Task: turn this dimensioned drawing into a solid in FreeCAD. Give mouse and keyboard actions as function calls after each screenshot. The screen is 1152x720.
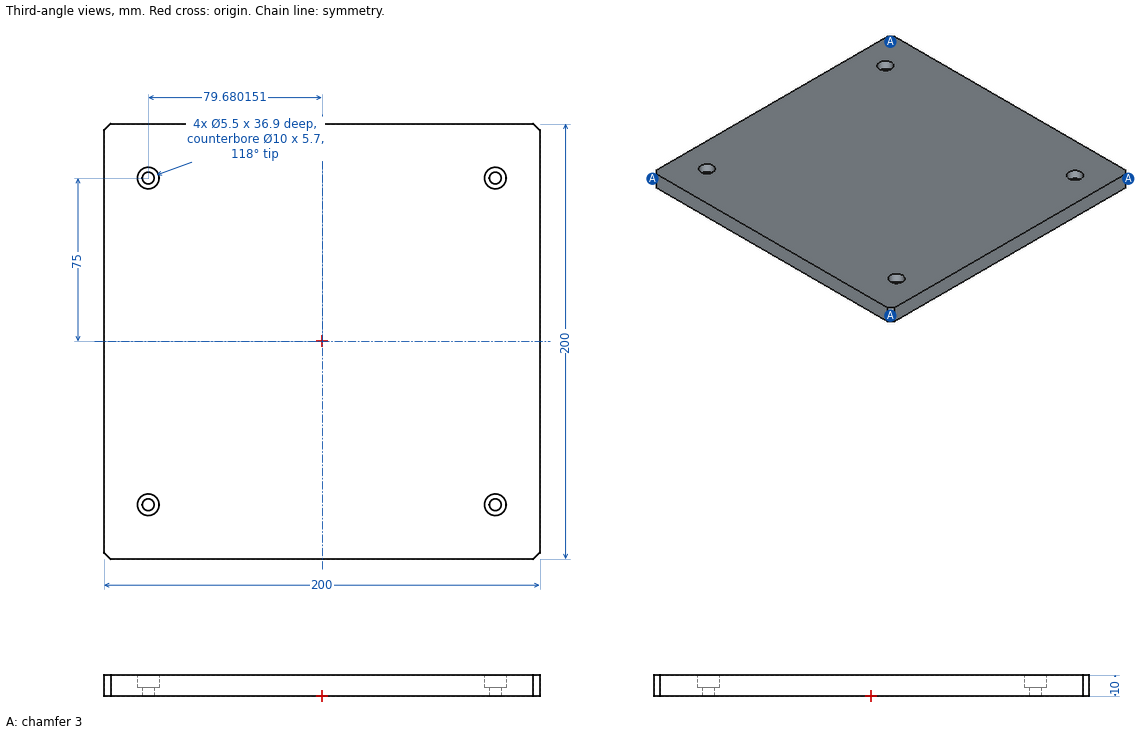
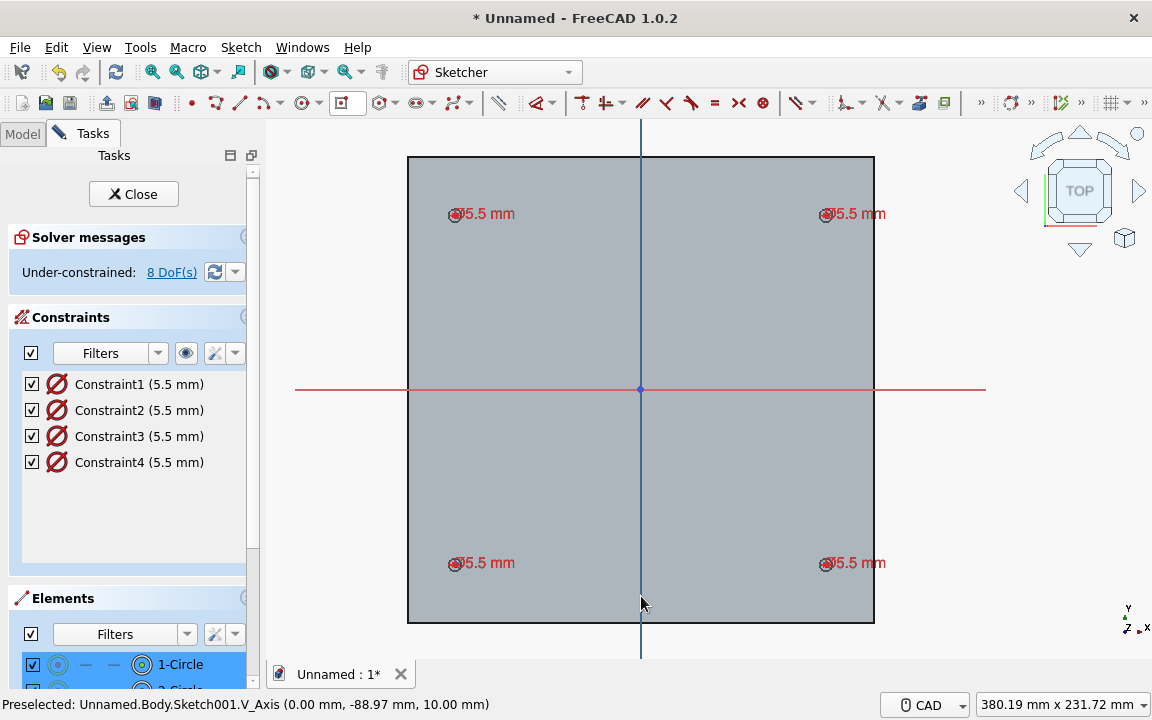
key(s)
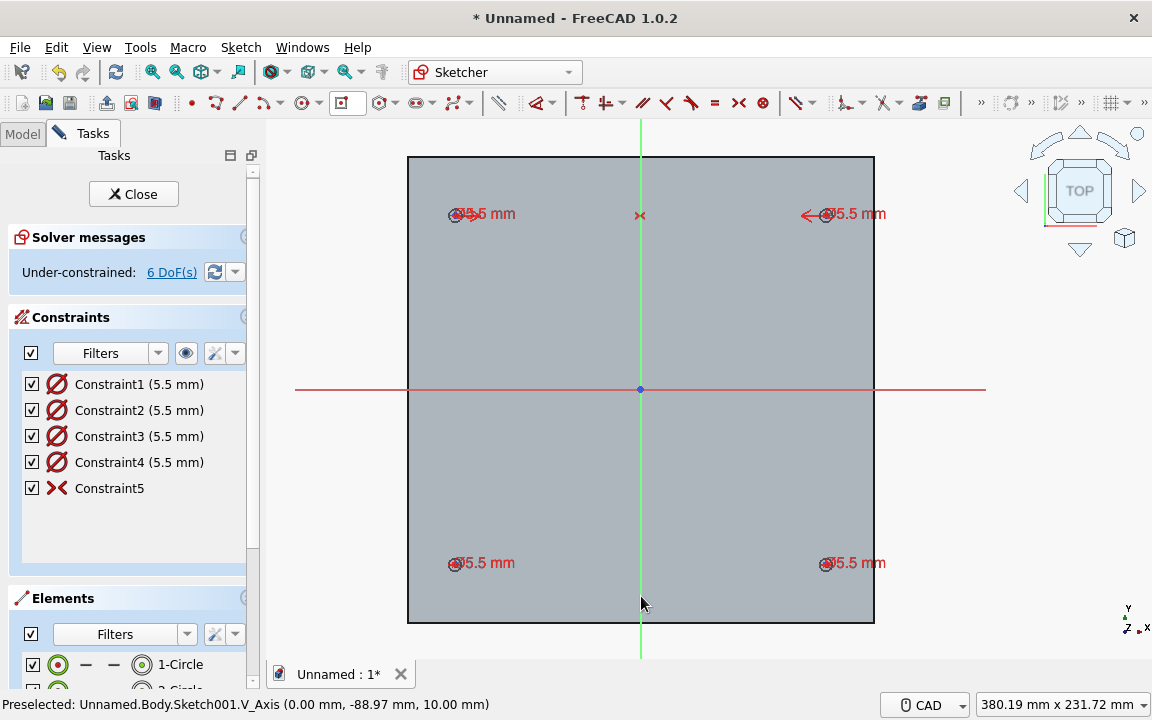
click(826, 216)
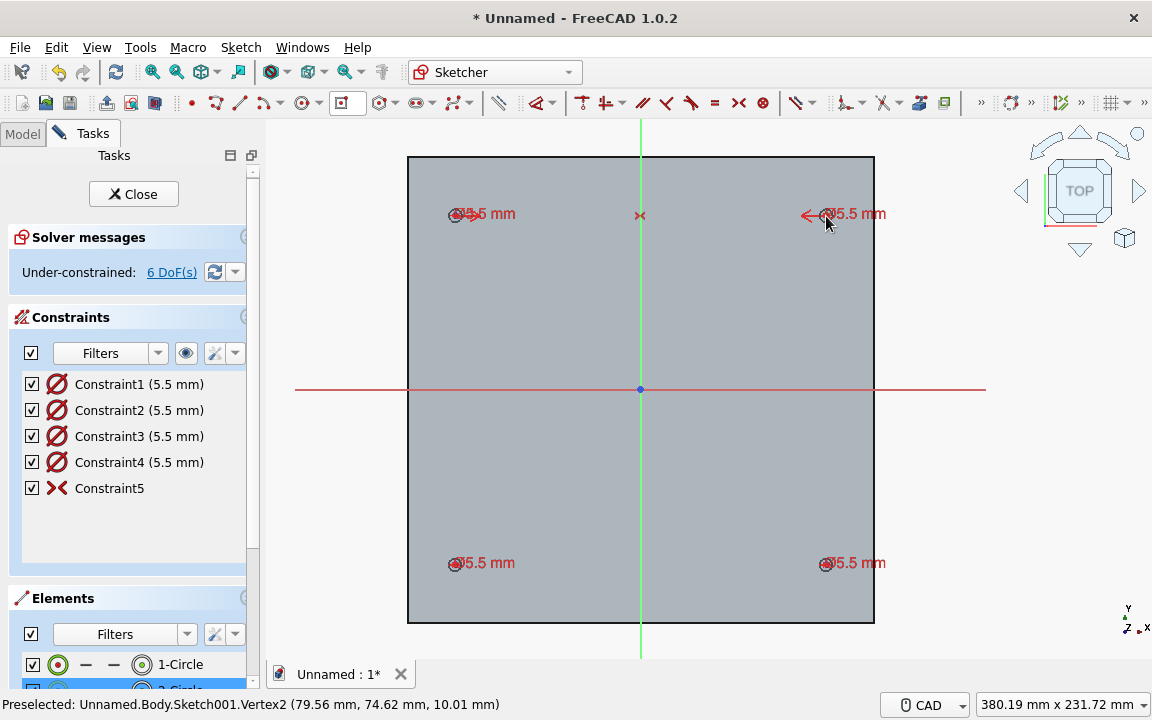
click(826, 565)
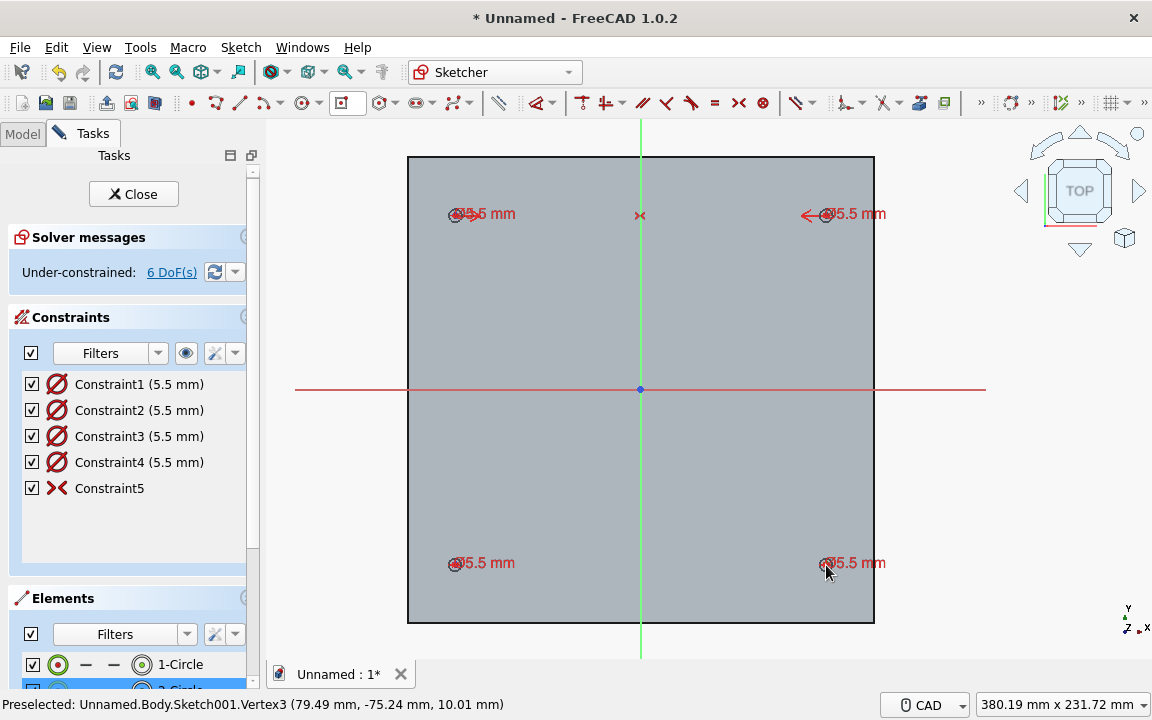
click(344, 390)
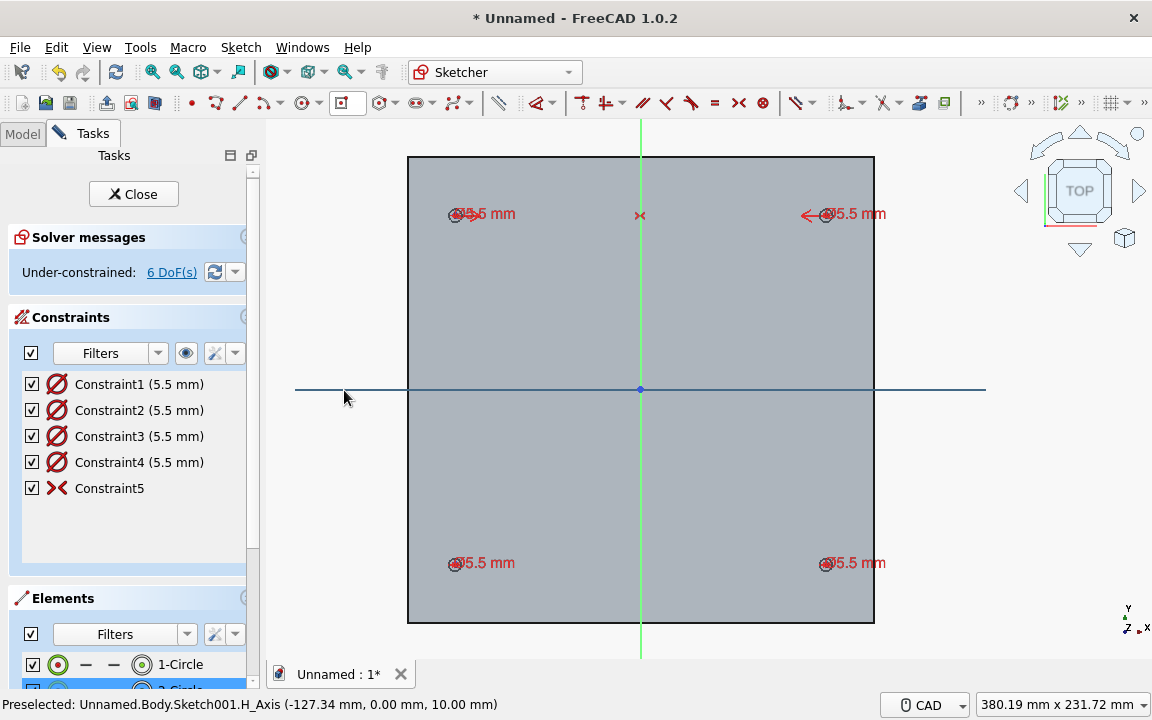
click(740, 104)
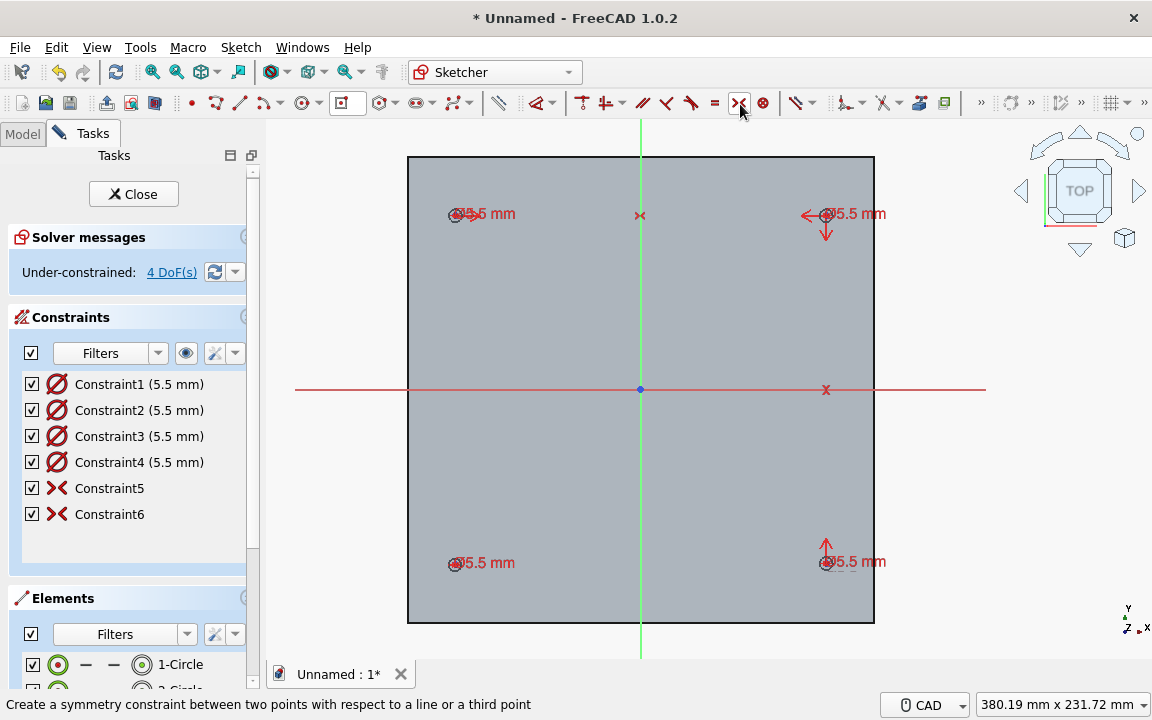
click(455, 216)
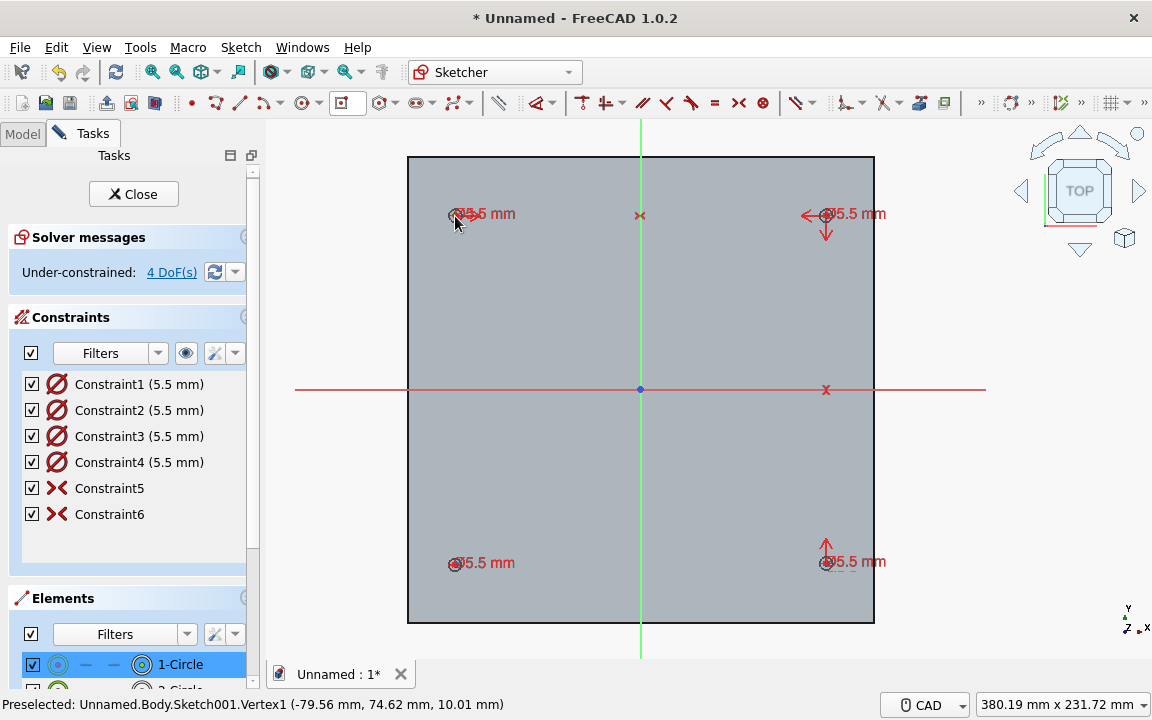
click(455, 565)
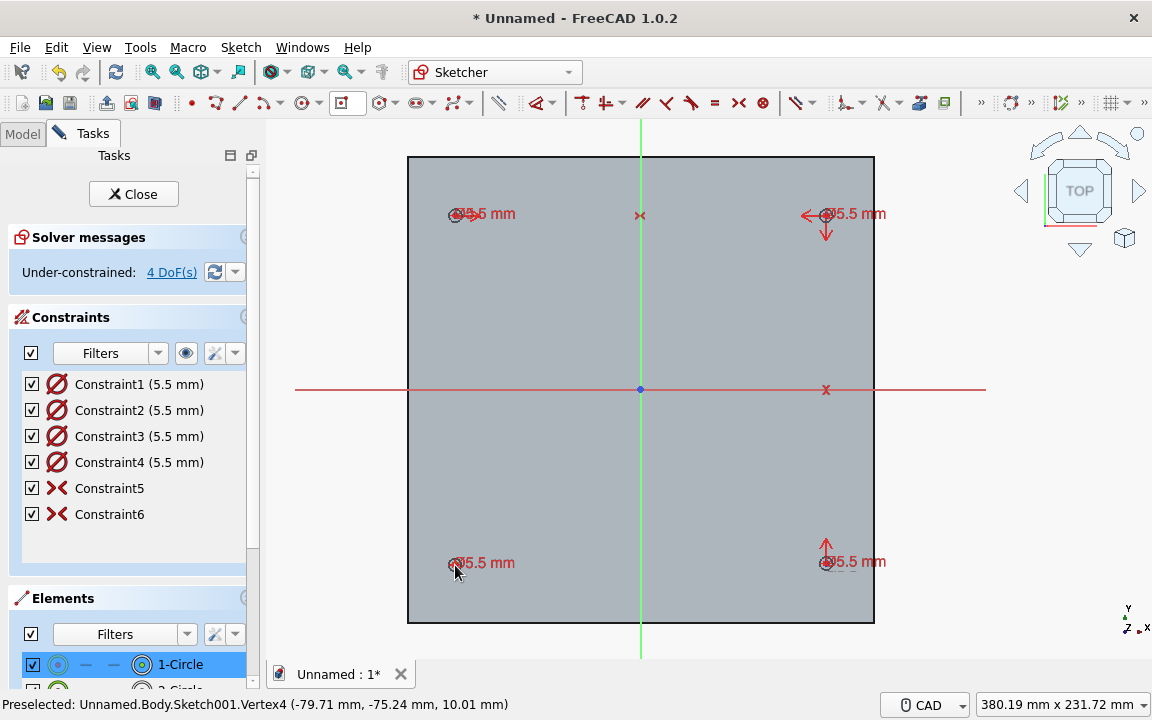
click(344, 390)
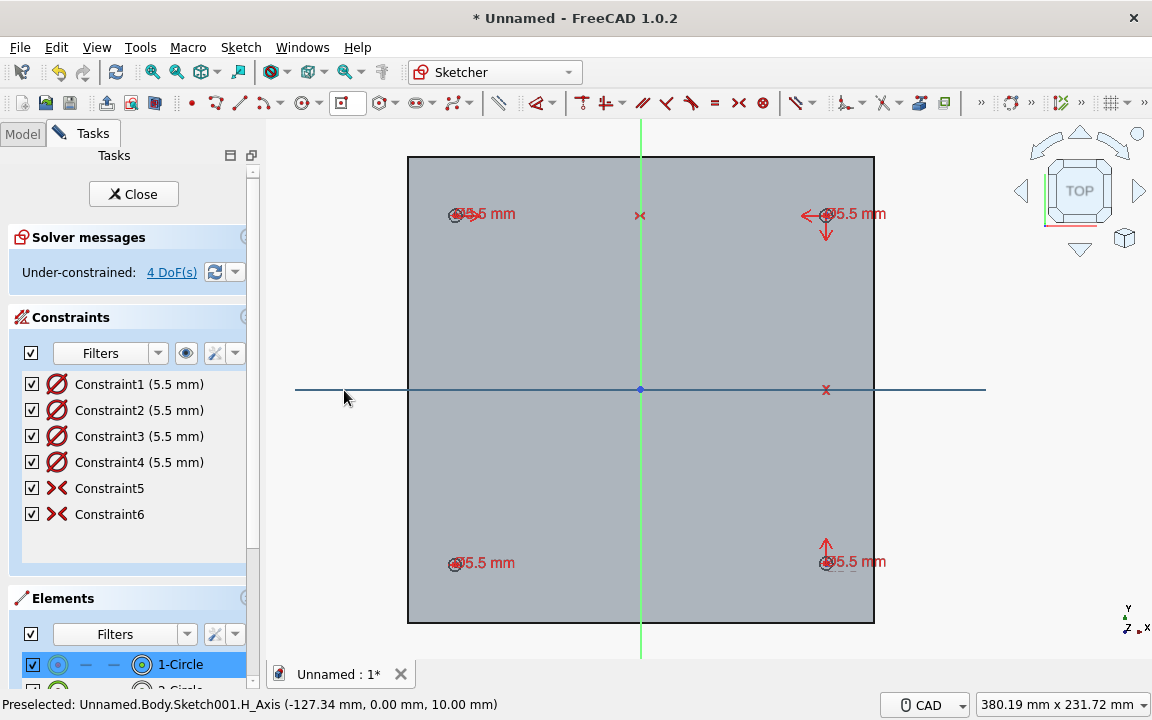
click(740, 104)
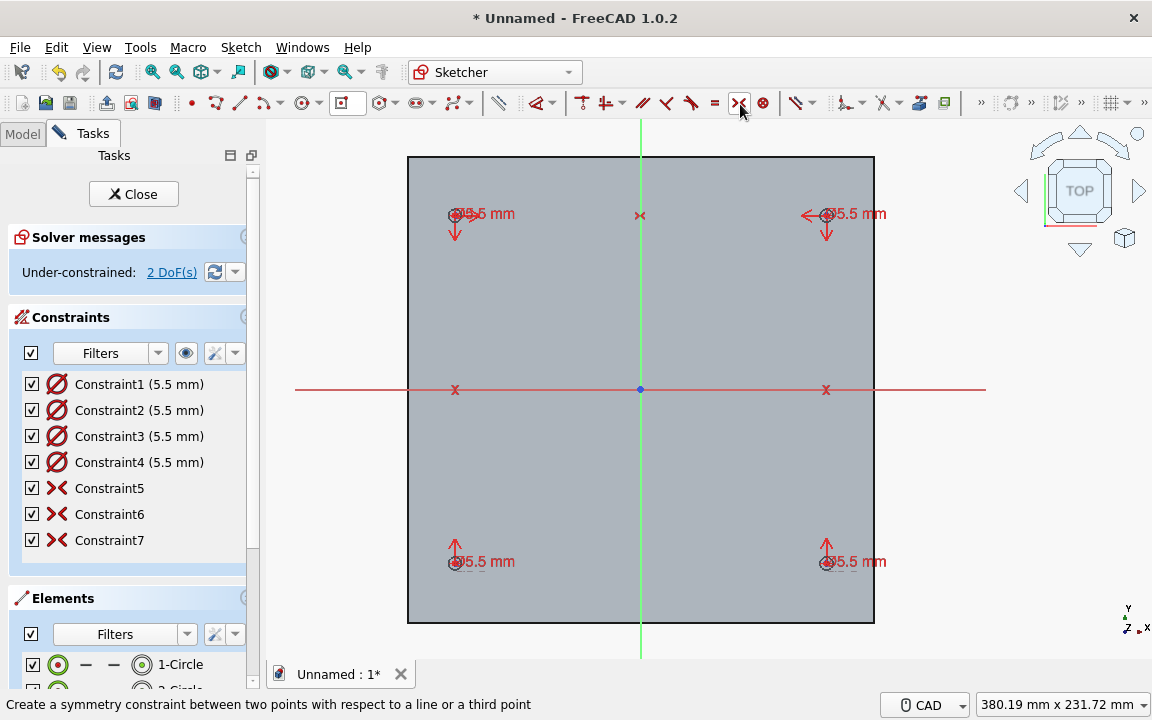
click(455, 216)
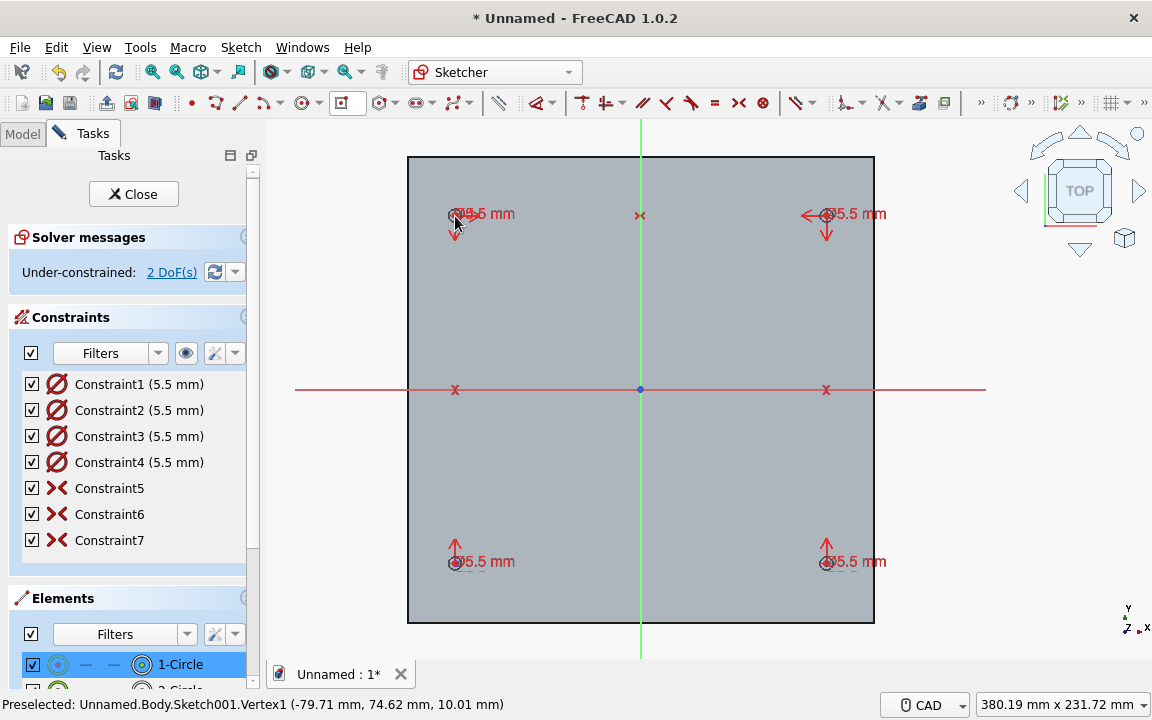
click(554, 104)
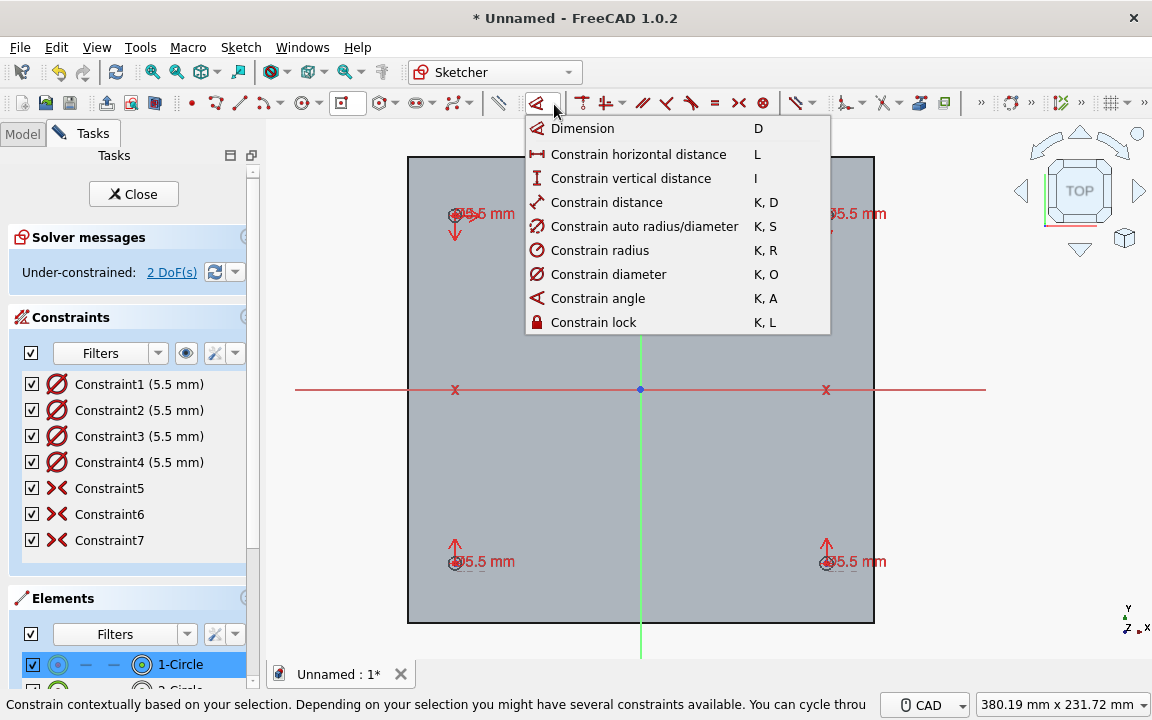
click(678, 178)